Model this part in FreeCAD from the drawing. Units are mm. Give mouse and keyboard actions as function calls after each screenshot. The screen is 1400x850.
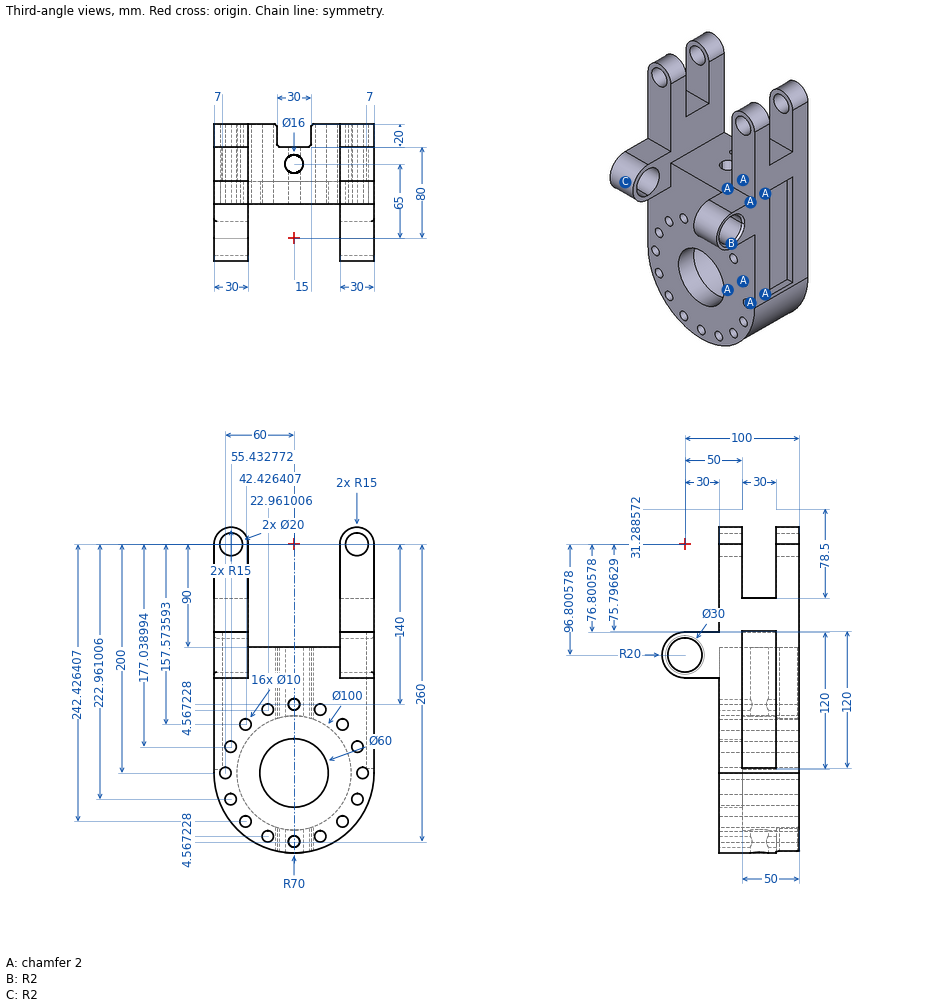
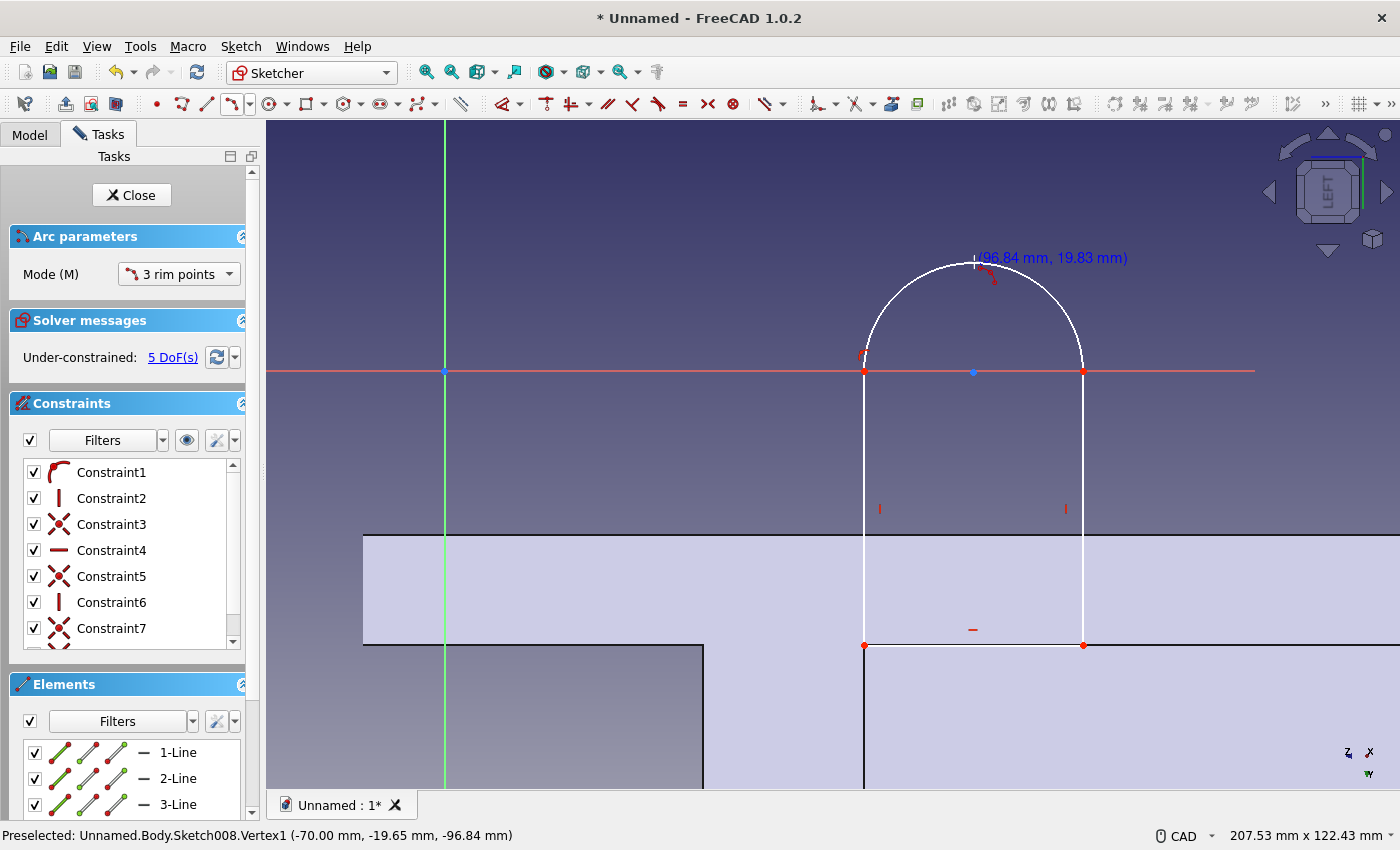
click(268, 104)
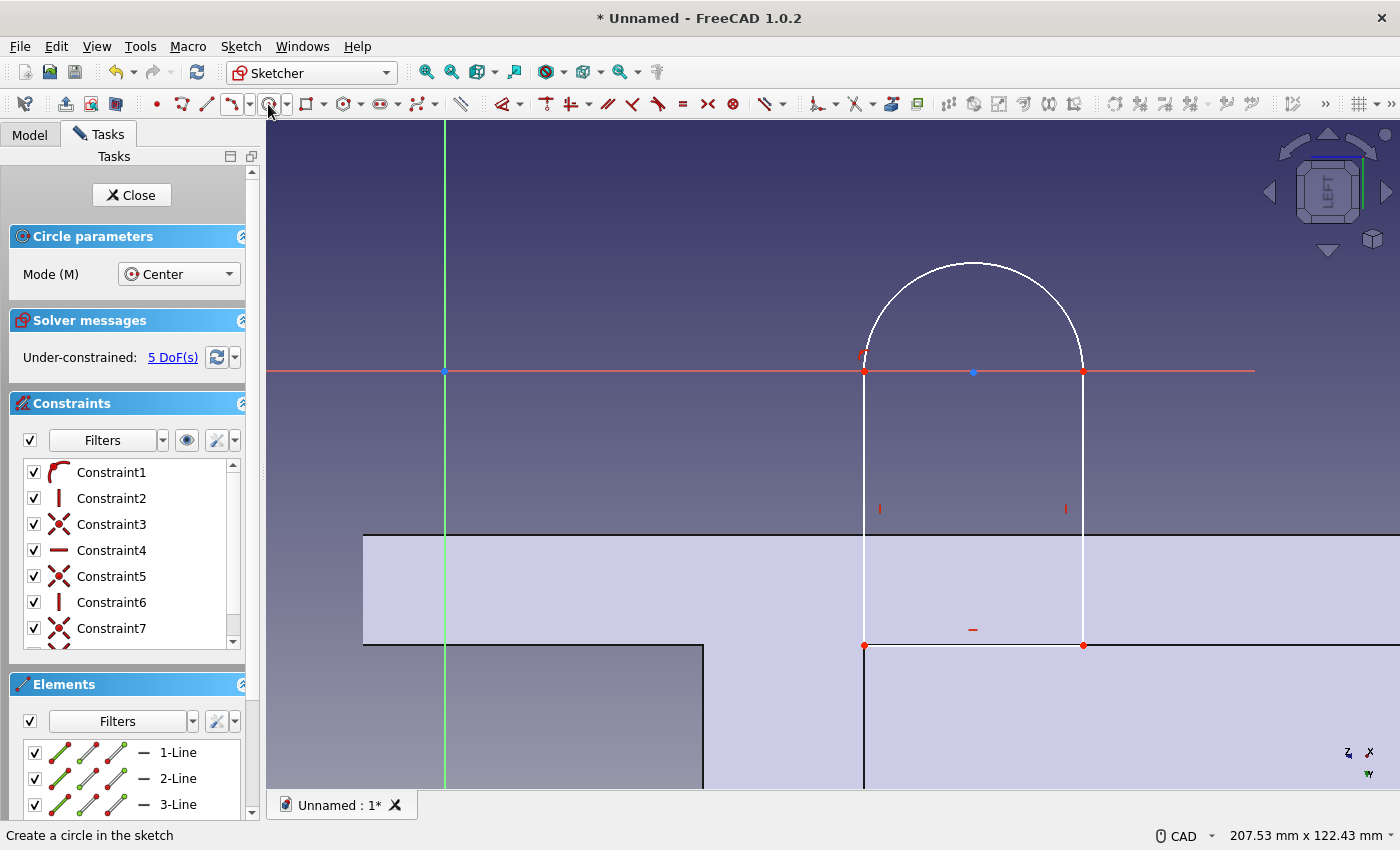
click(974, 371)
click(1032, 313)
key(Escape)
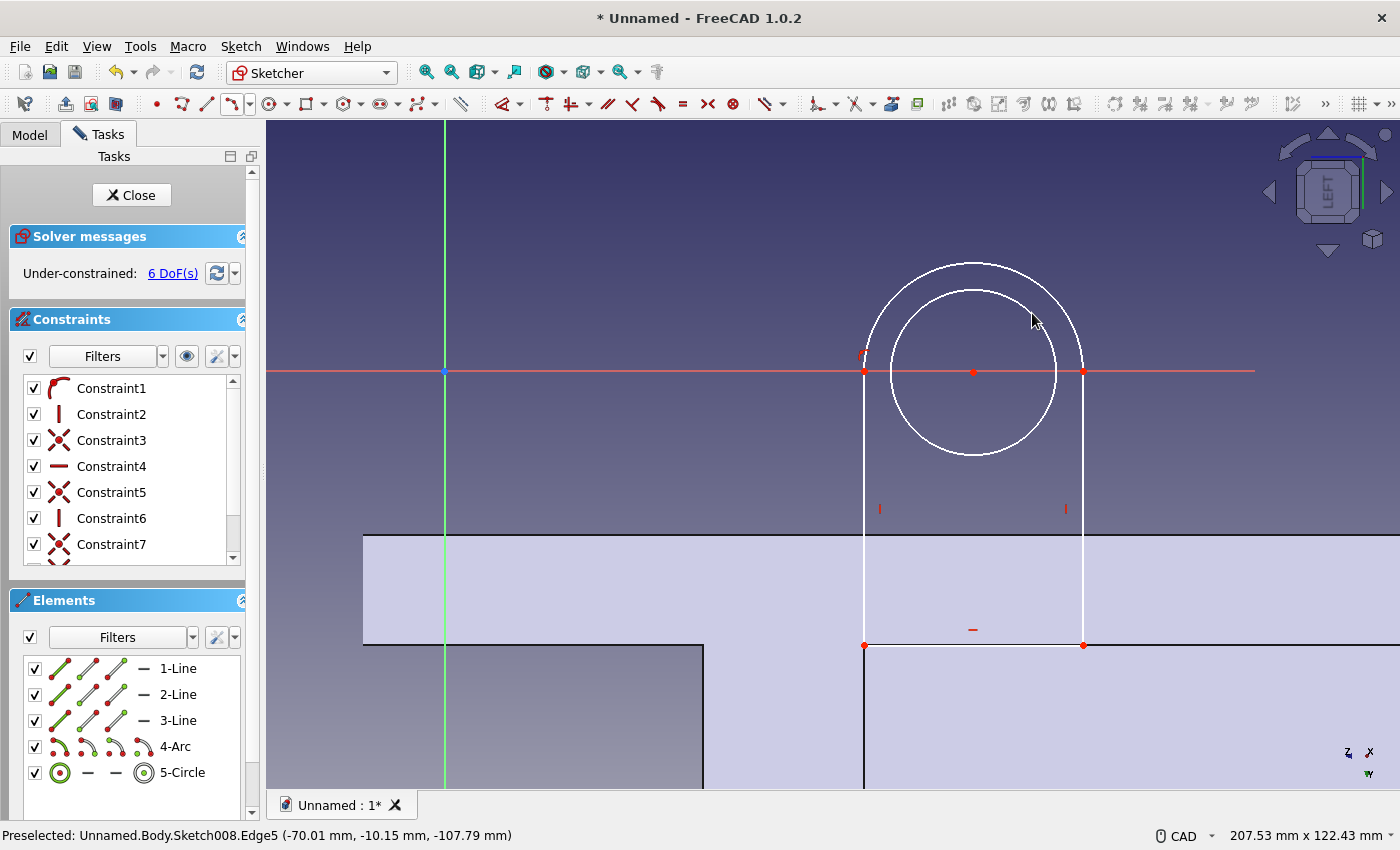
click(864, 454)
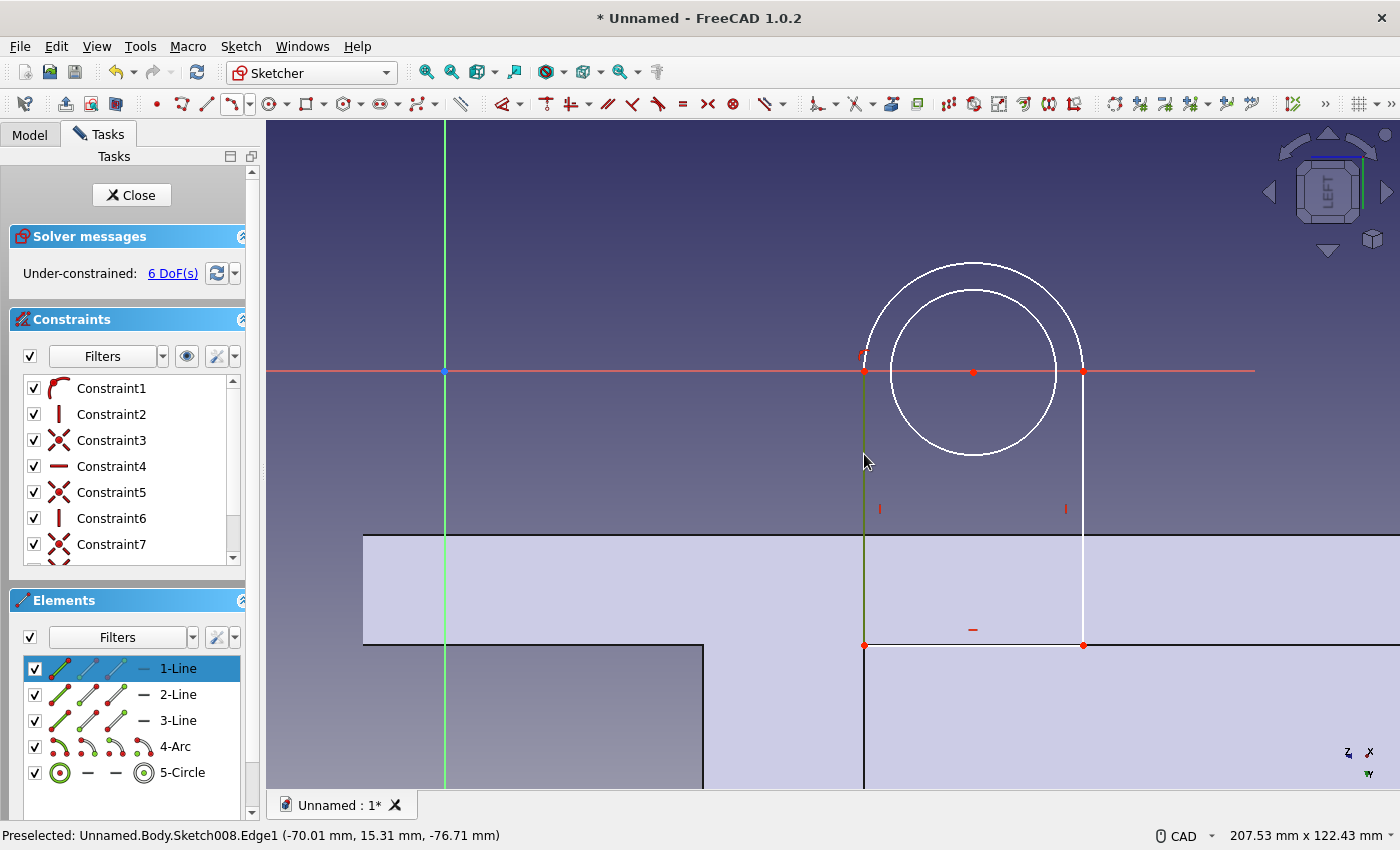
click(1037, 284)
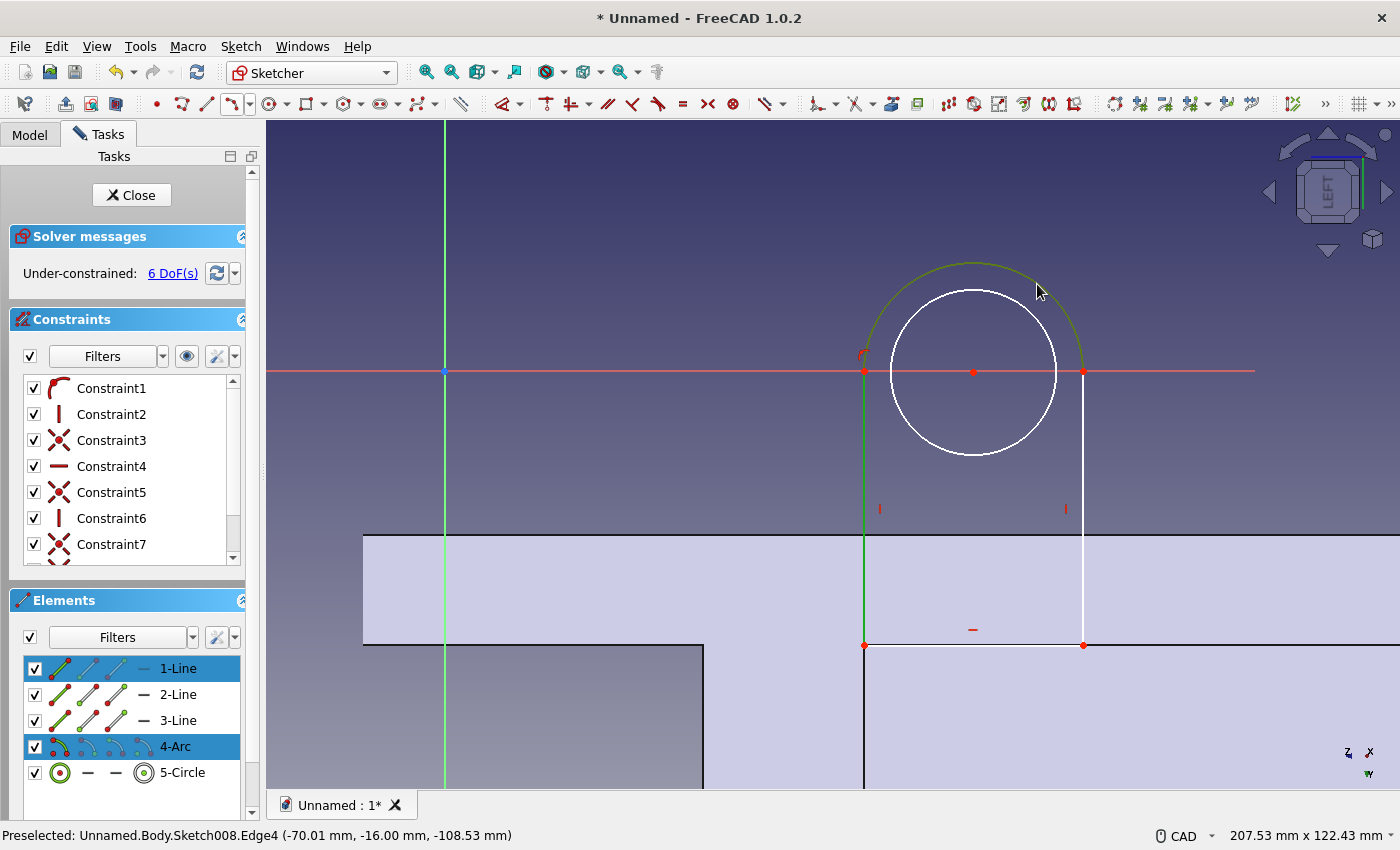
key(t)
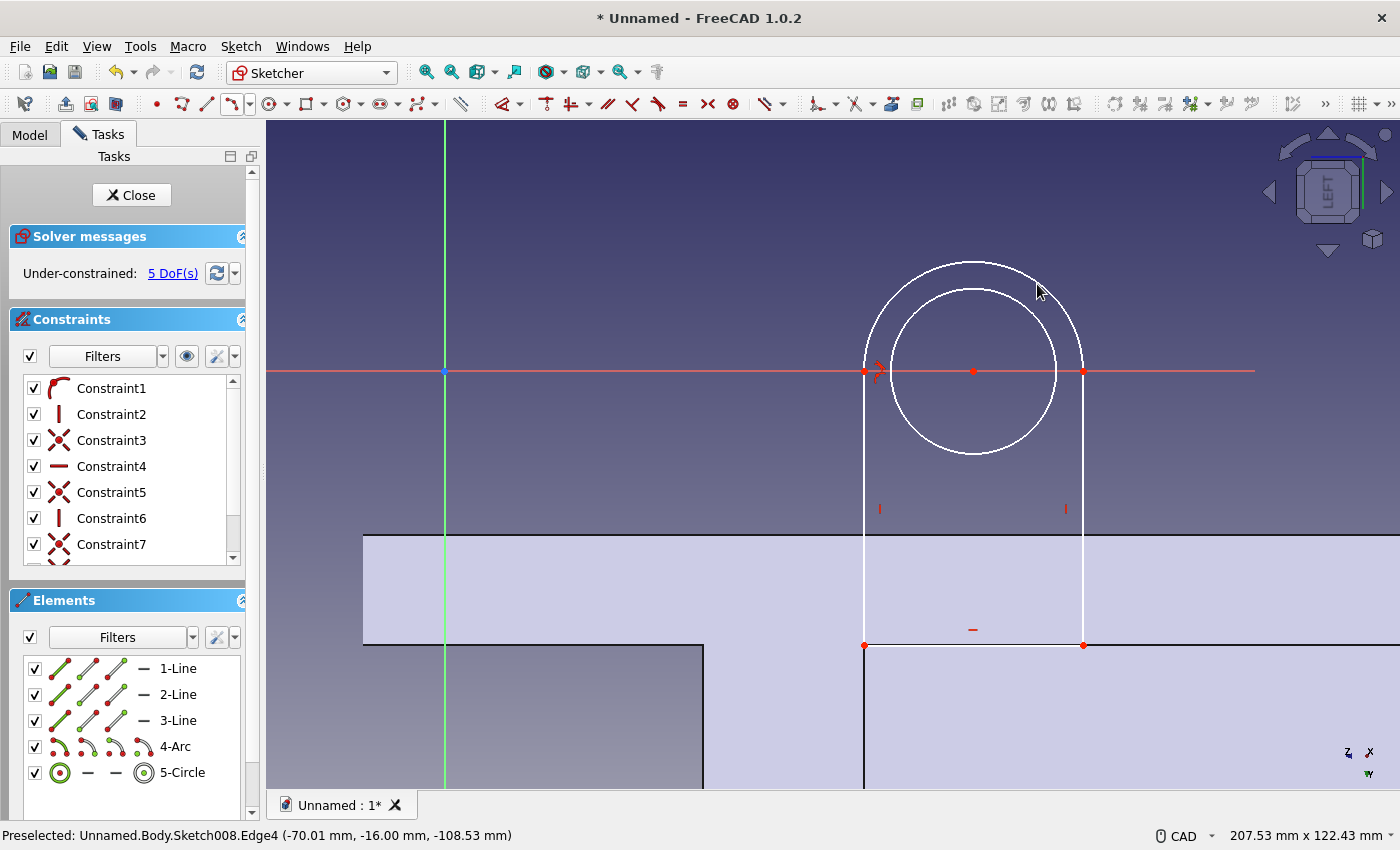
click(1083, 564)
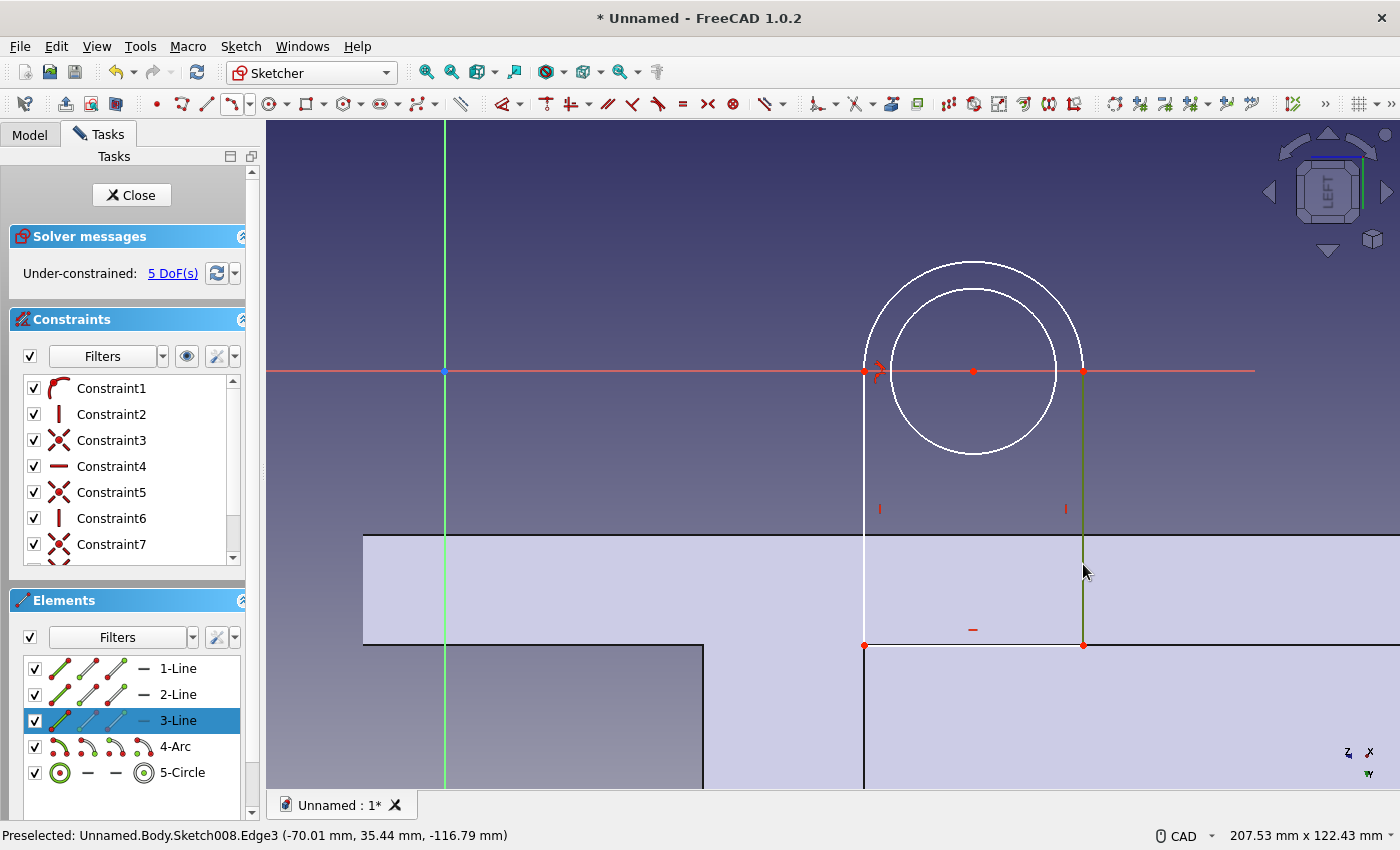
click(1038, 283)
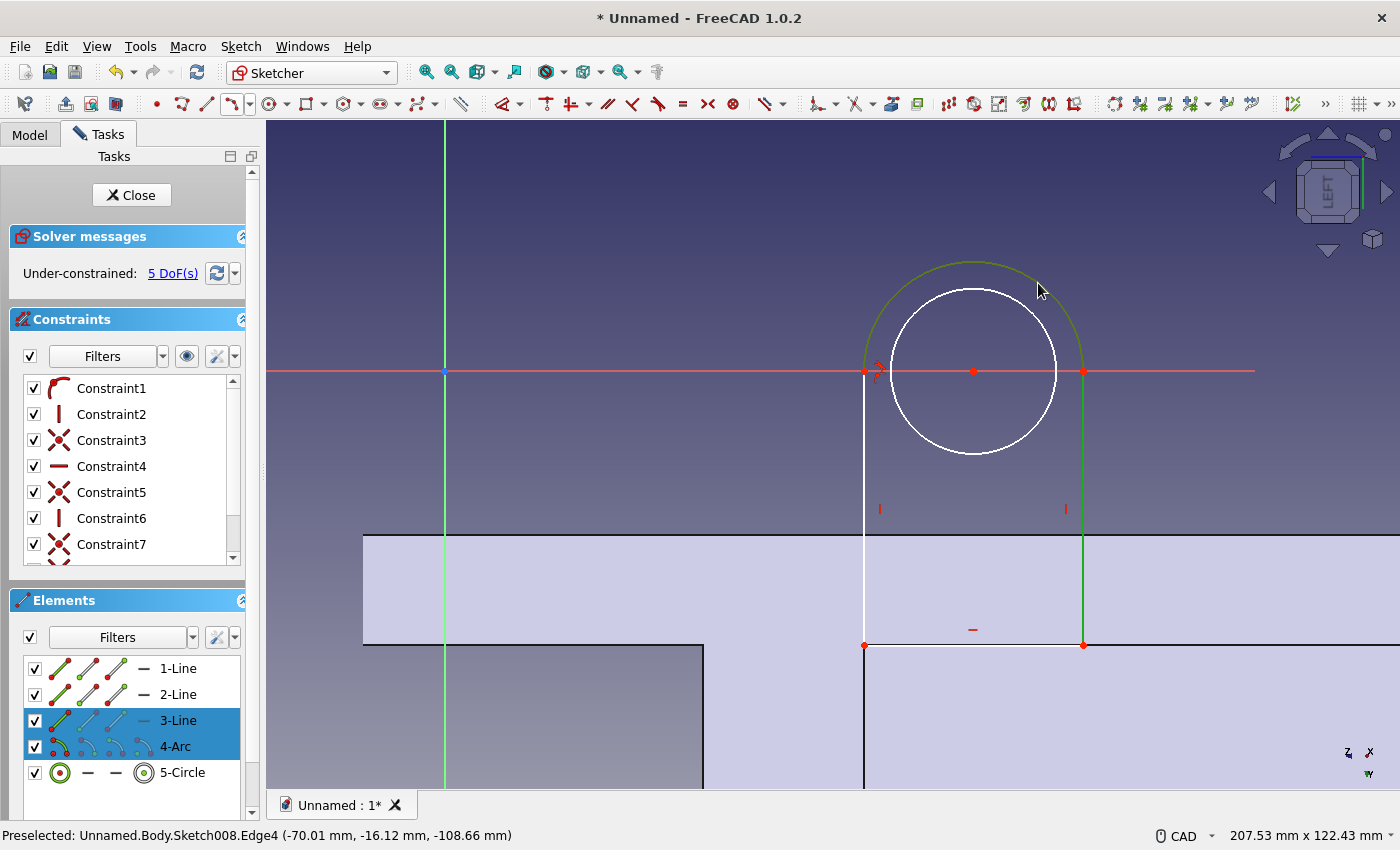
key(t)